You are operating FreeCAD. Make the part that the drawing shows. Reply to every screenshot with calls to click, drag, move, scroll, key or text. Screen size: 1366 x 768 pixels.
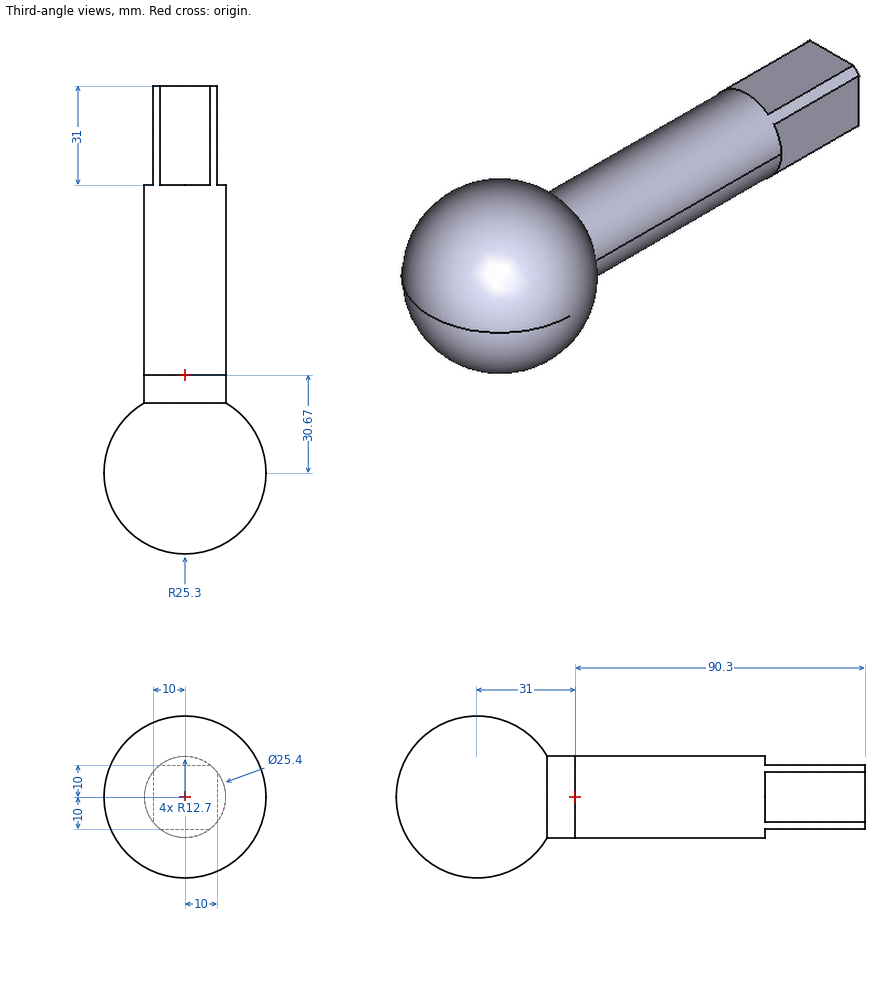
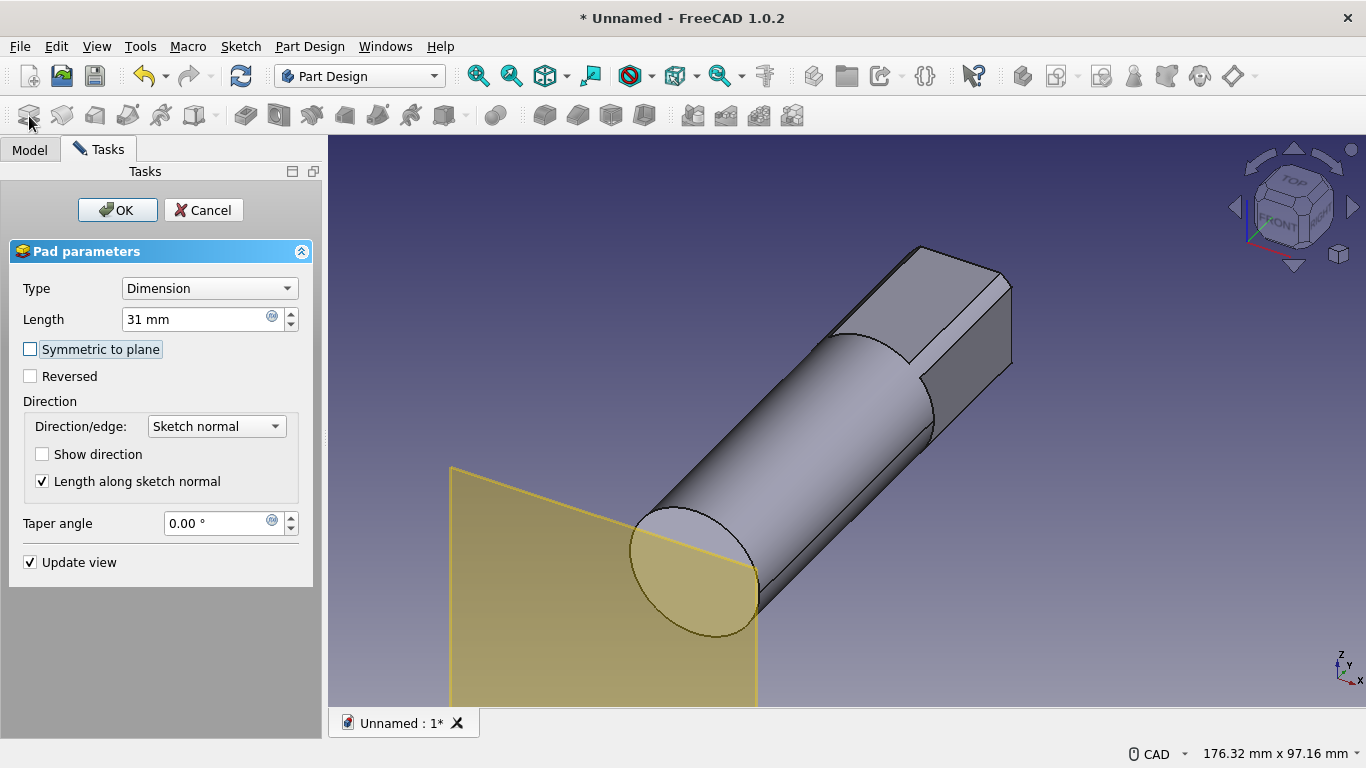
click(31, 376)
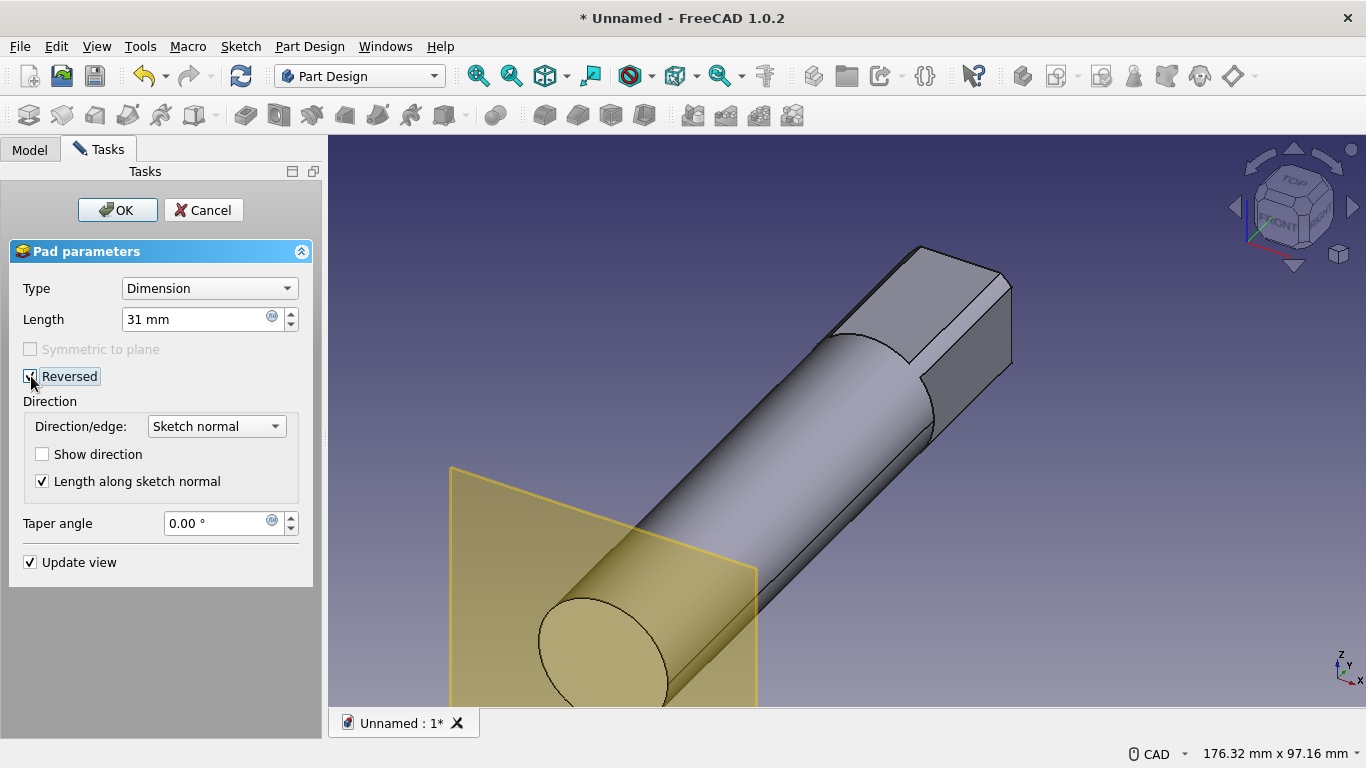
click(118, 210)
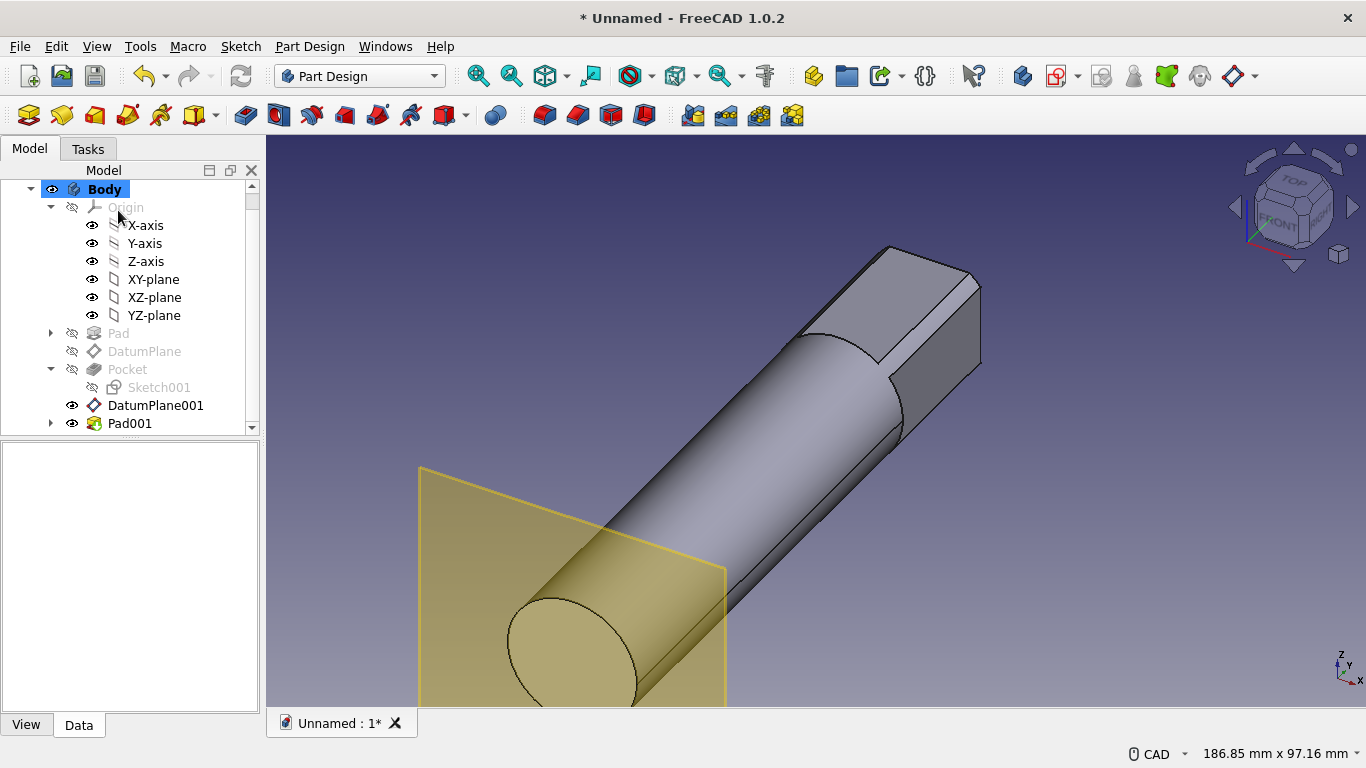
click(117, 405)
key(space)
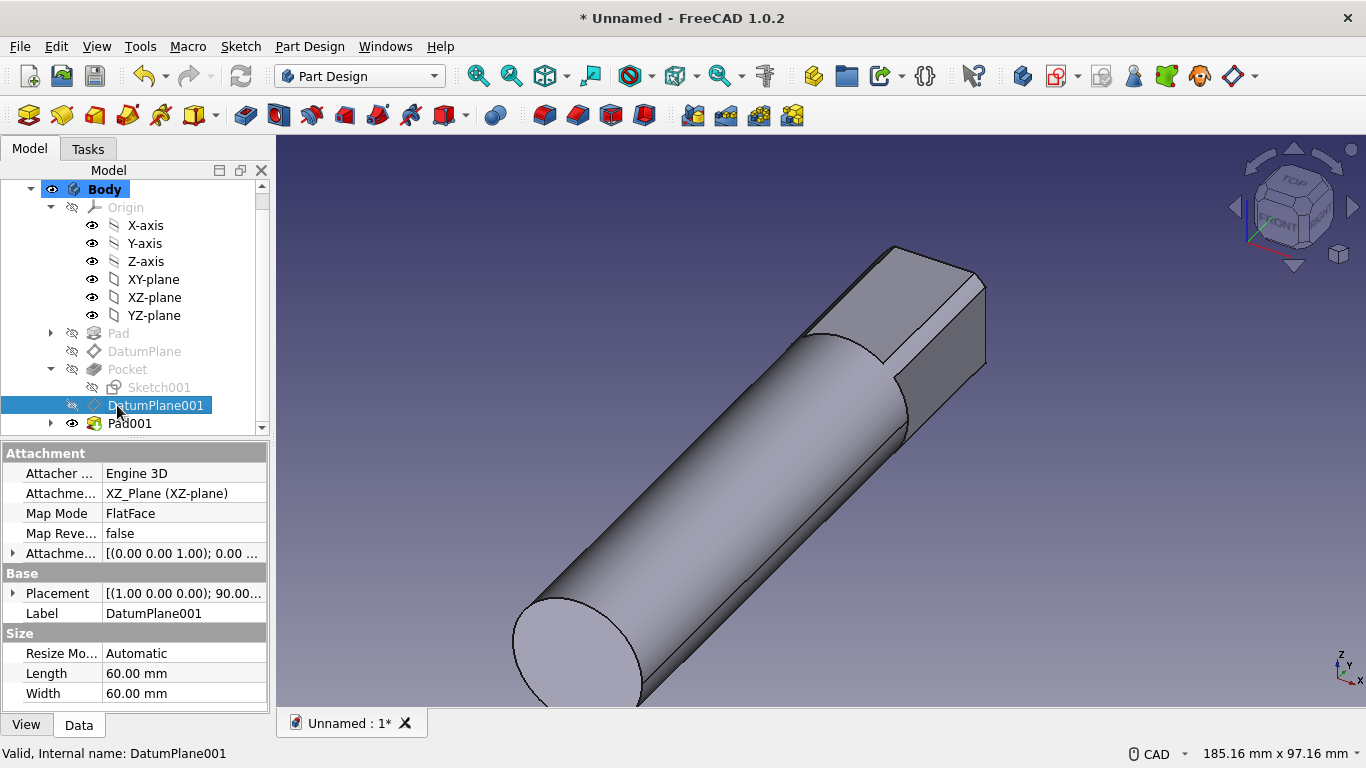
click(479, 76)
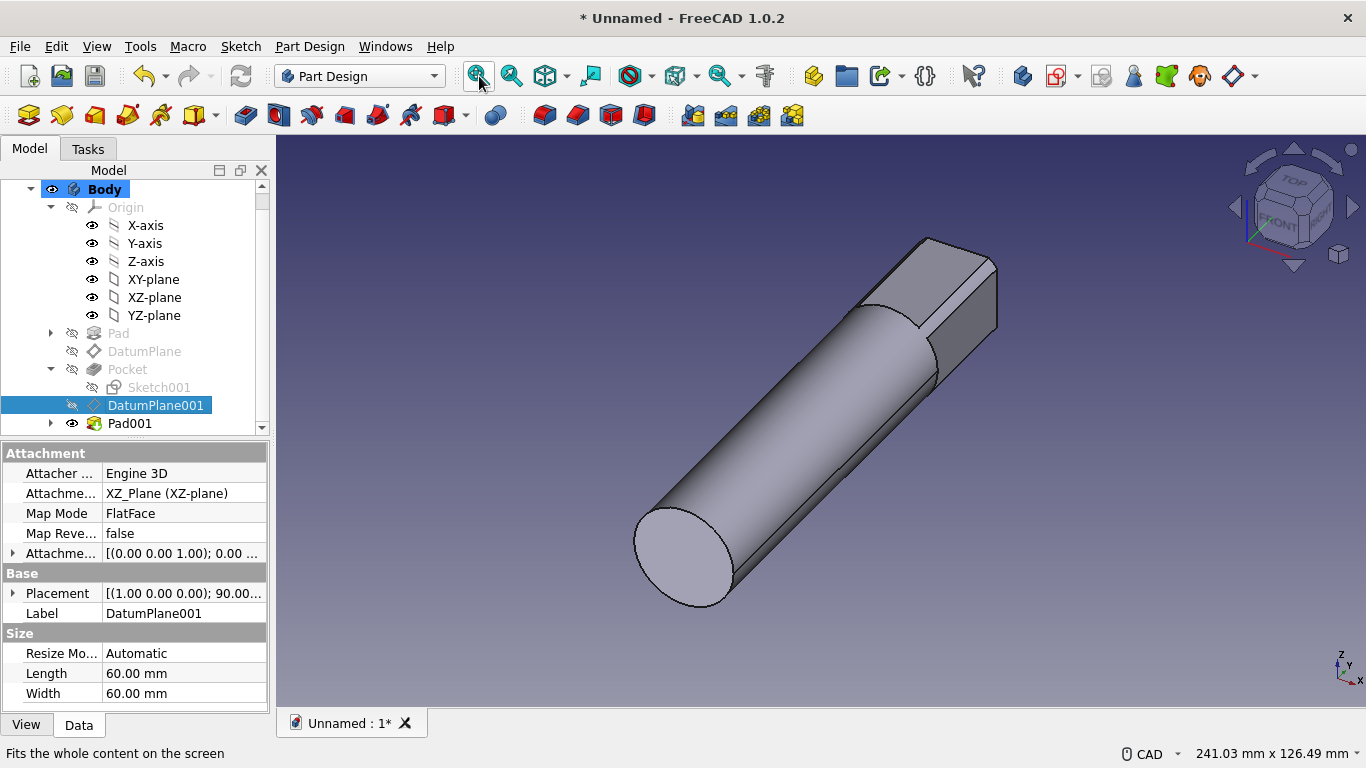
click(316, 667)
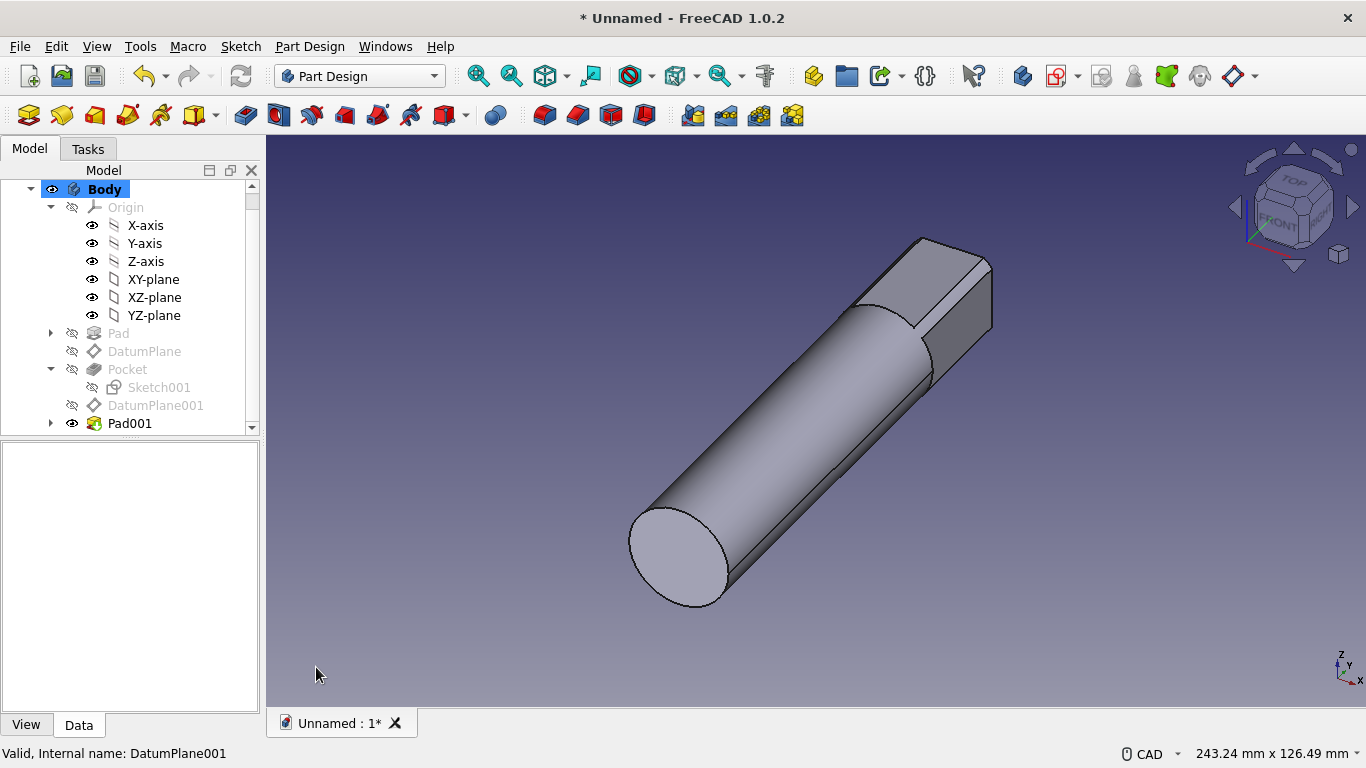
click(1023, 76)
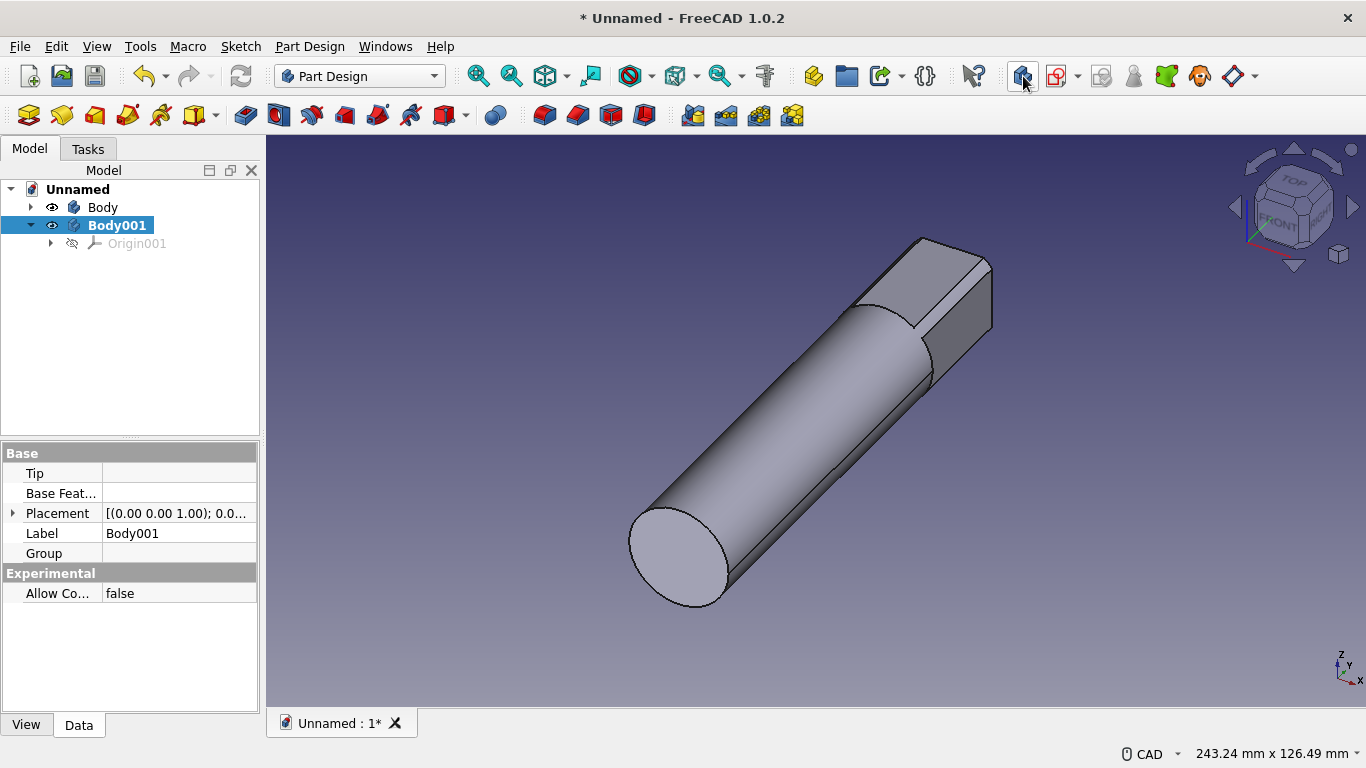
click(306, 667)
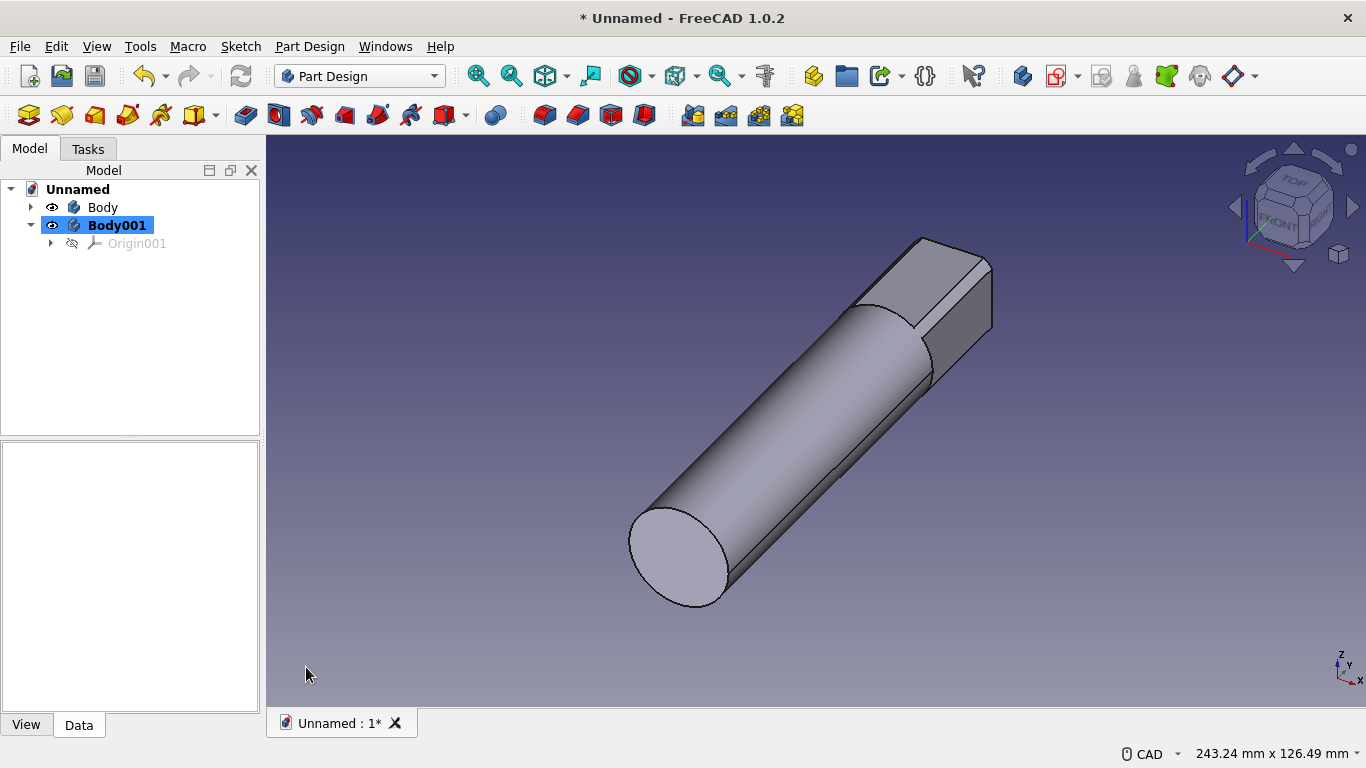
click(1056, 76)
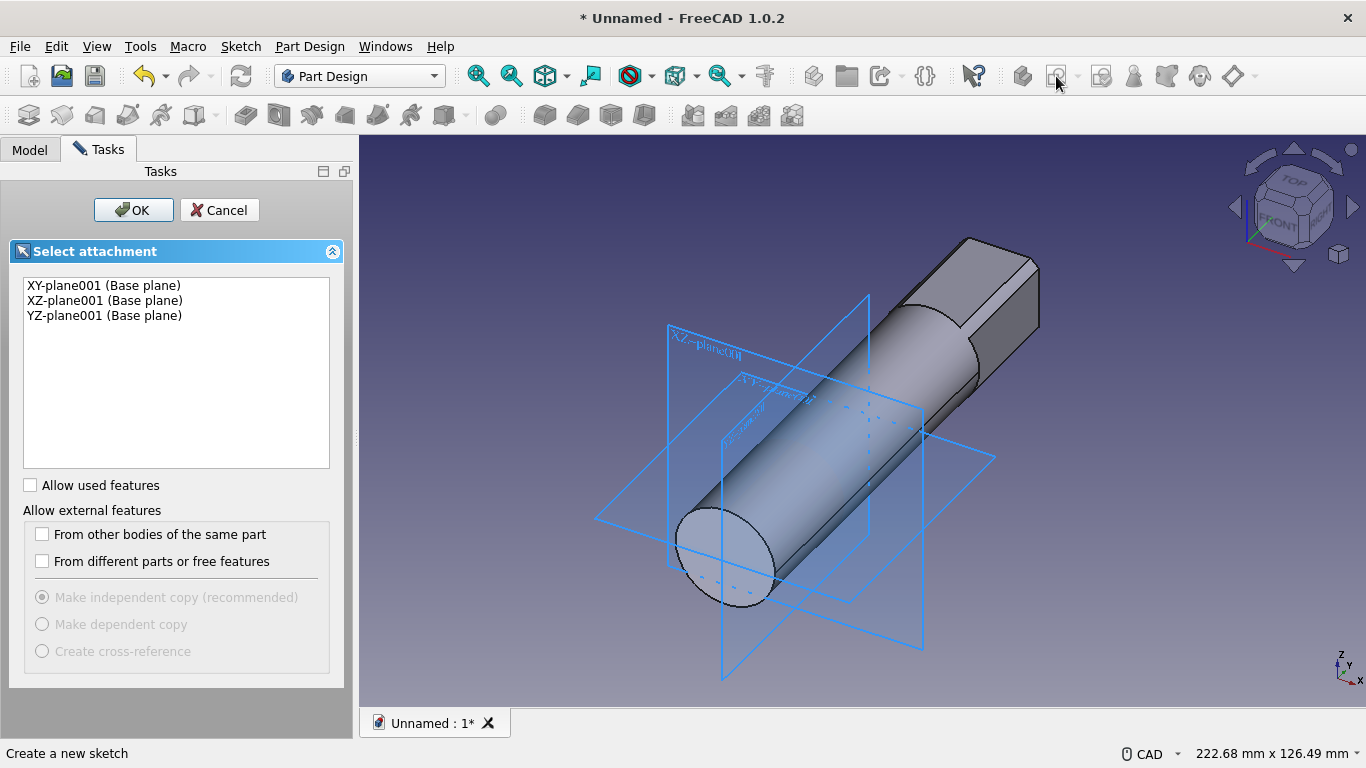
click(84, 286)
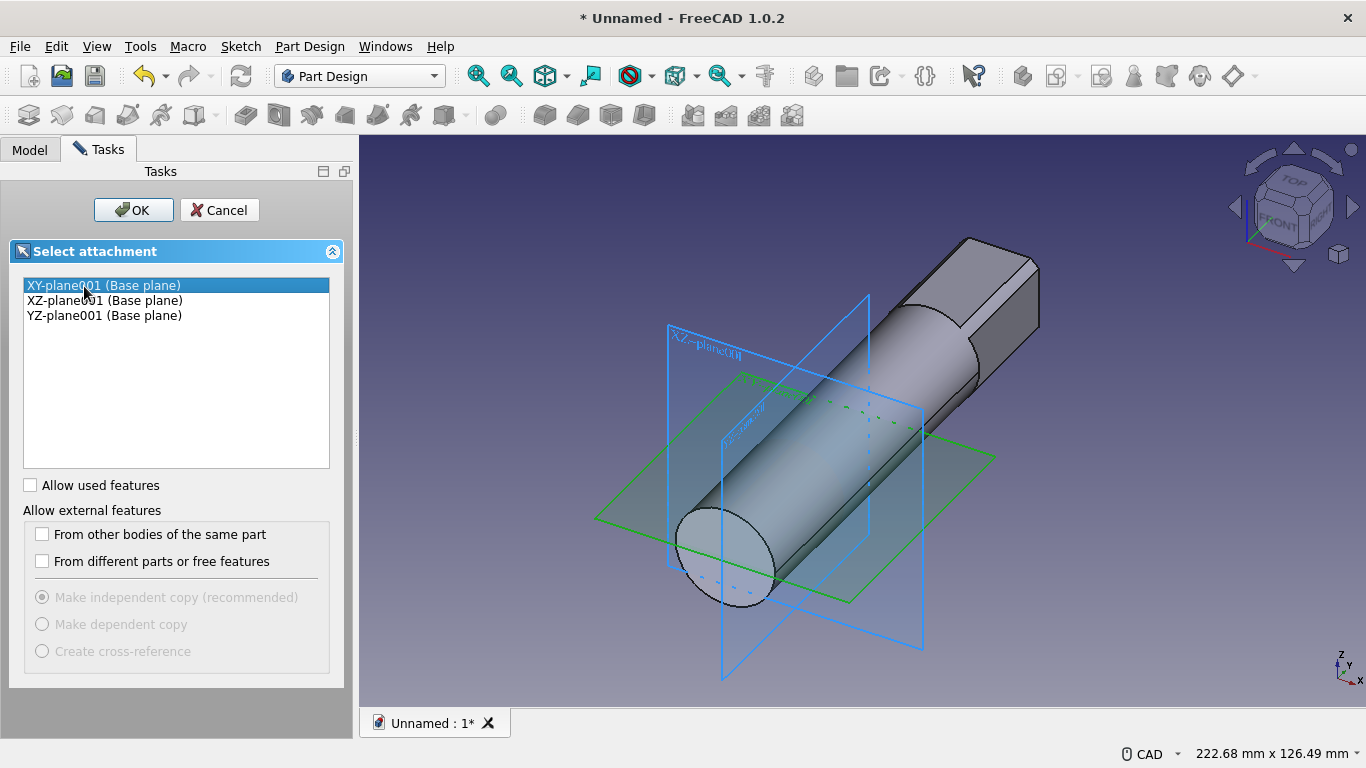
click(134, 210)